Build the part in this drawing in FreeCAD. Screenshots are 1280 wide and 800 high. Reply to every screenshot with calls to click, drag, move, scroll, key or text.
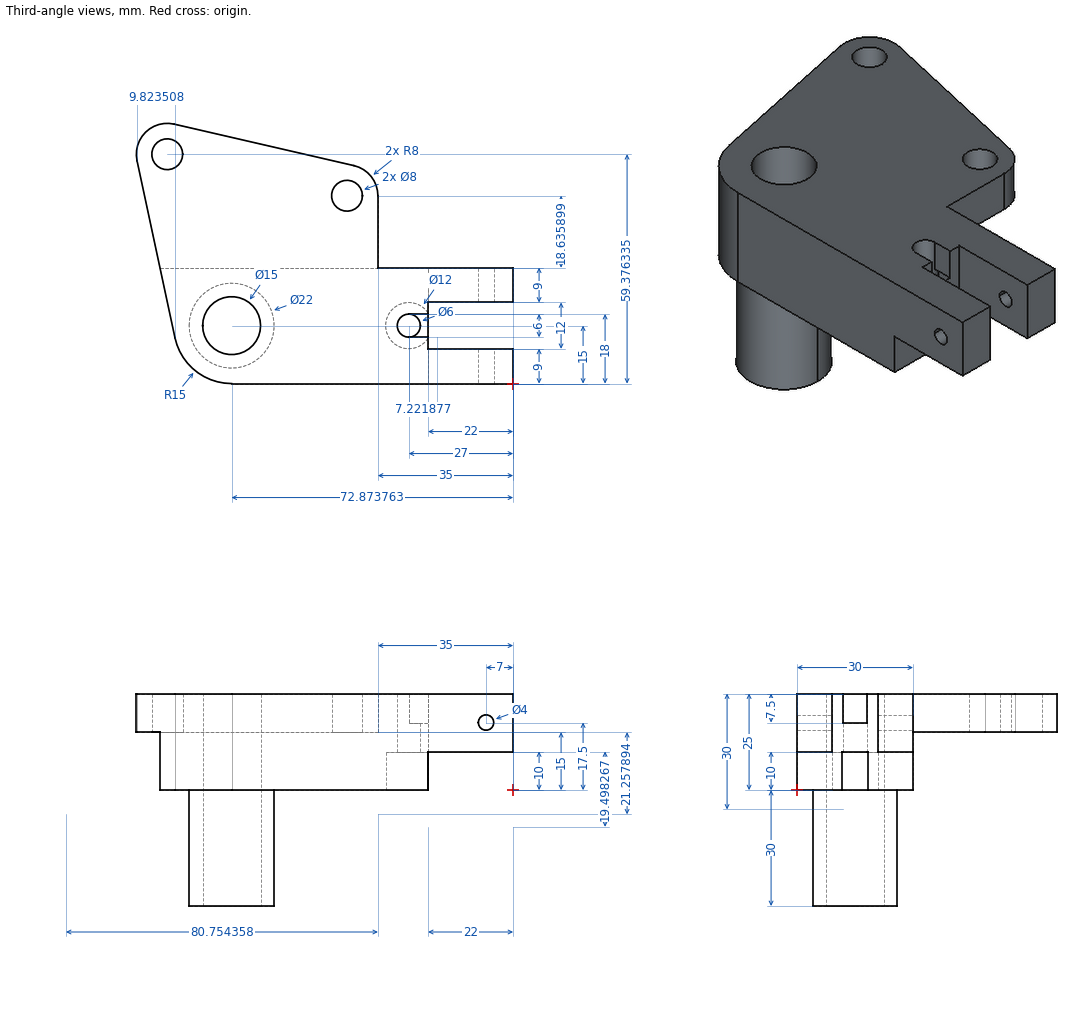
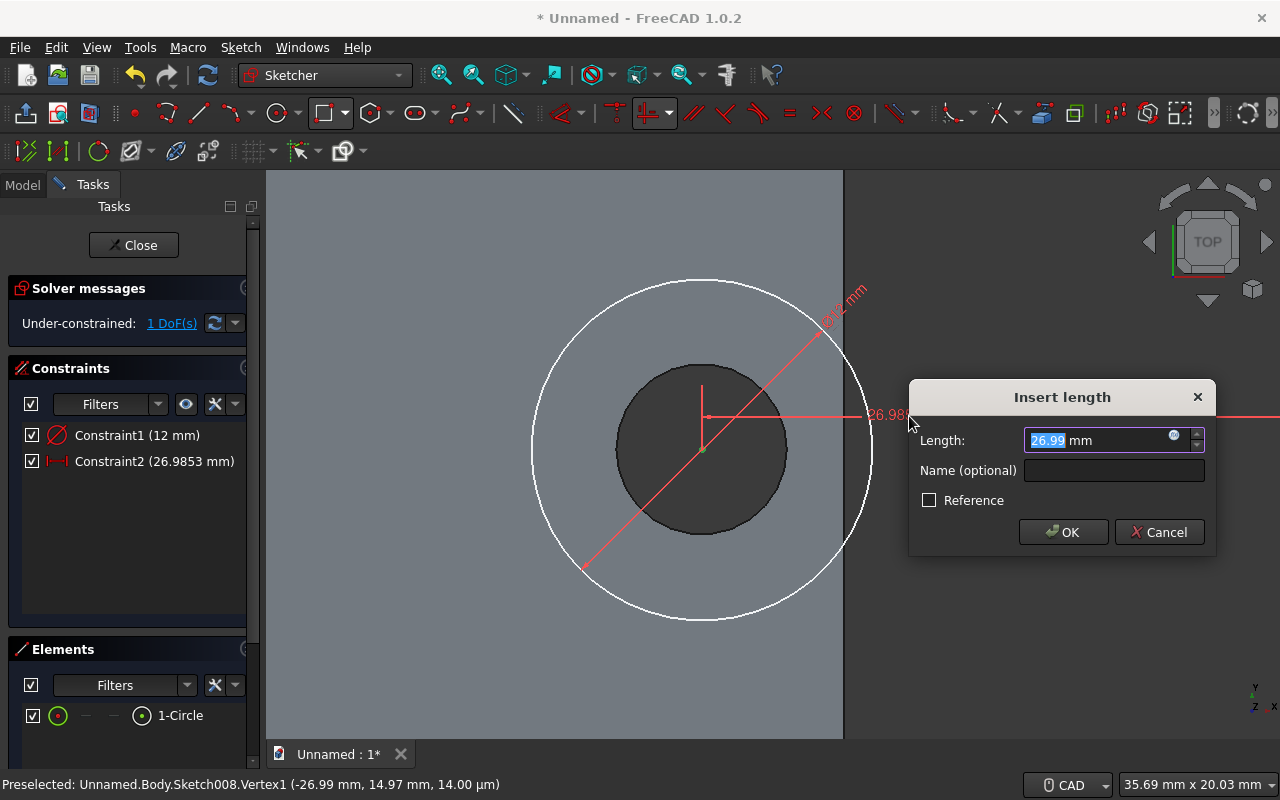
text(27)
key(Return)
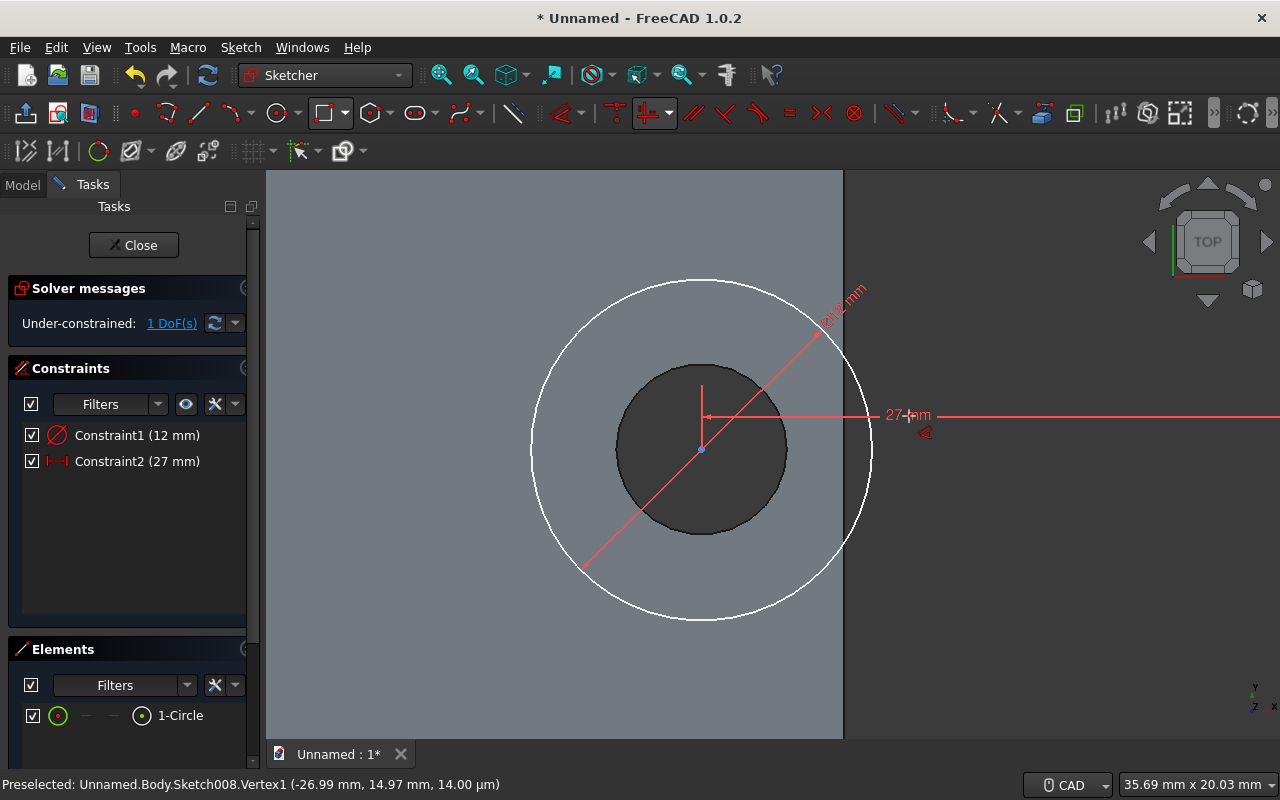
click(702, 450)
click(668, 581)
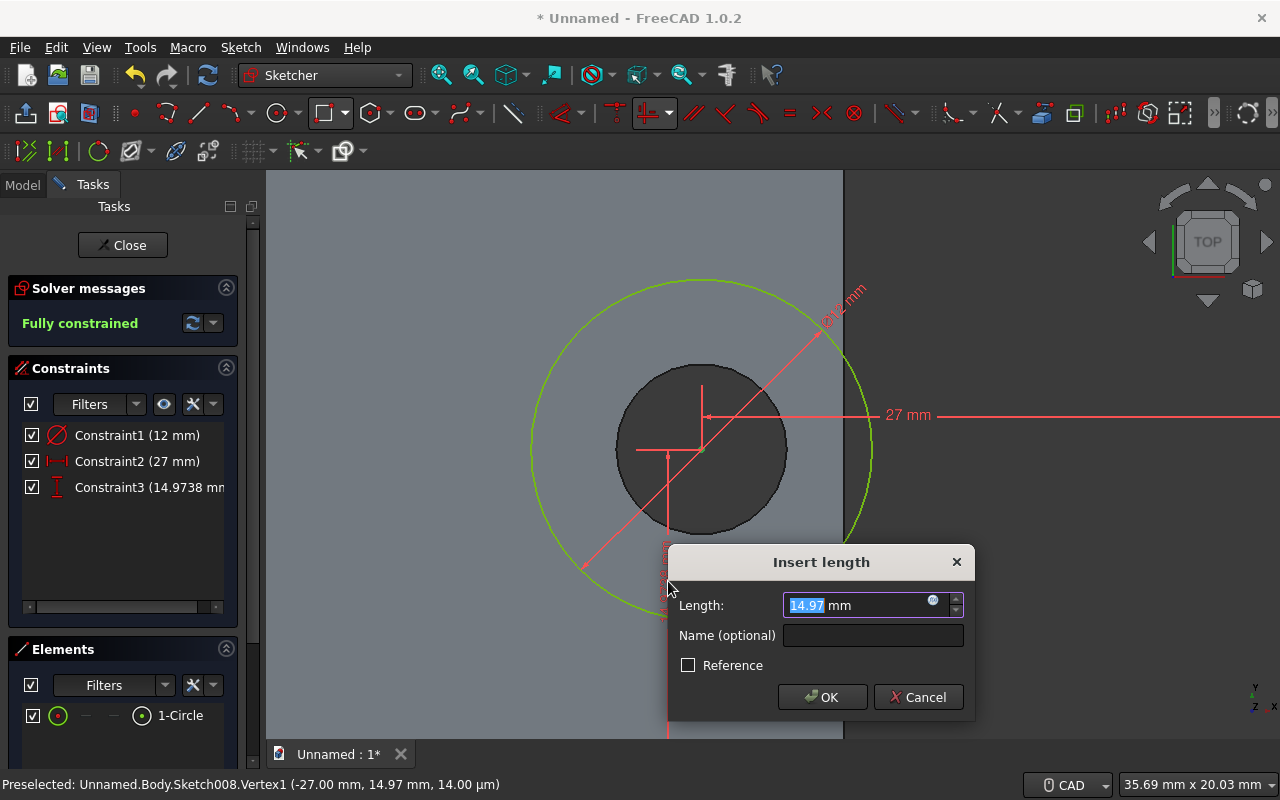
text(15)
key(Return)
key(Escape)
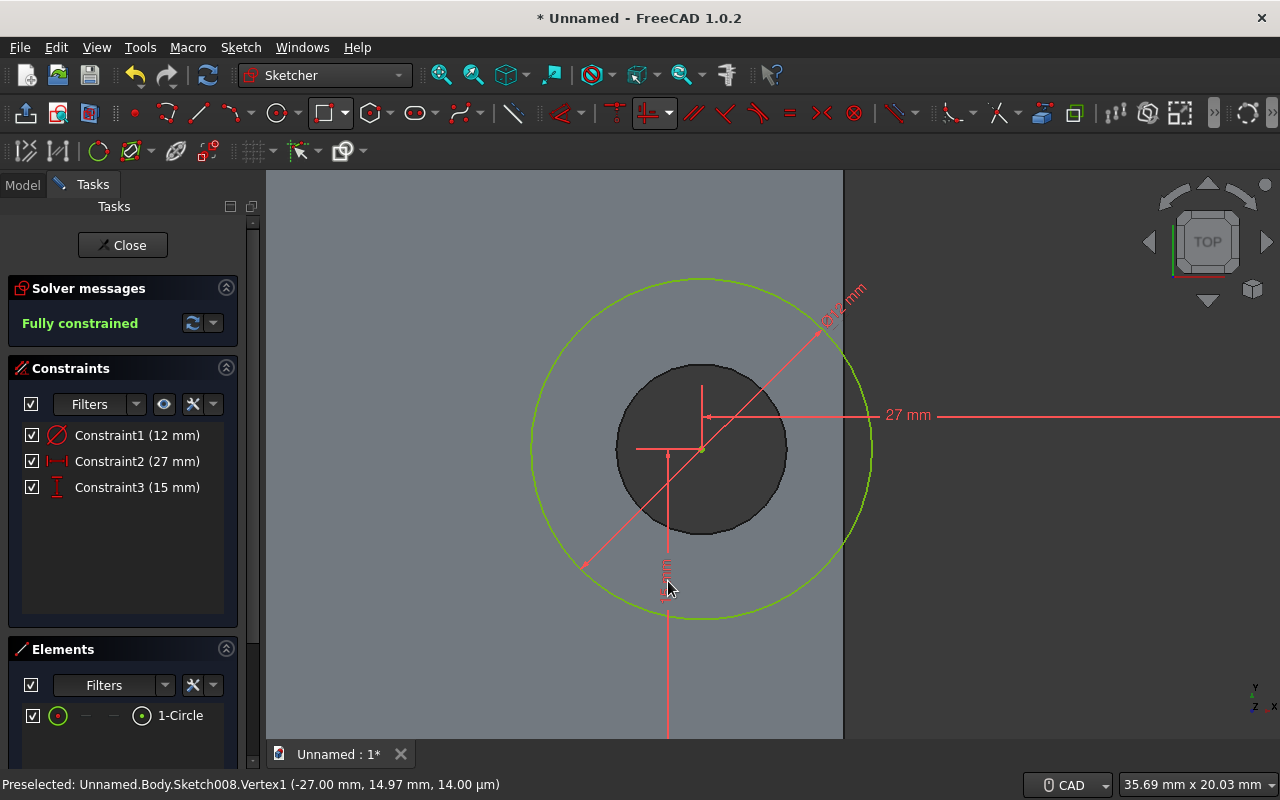
click(123, 245)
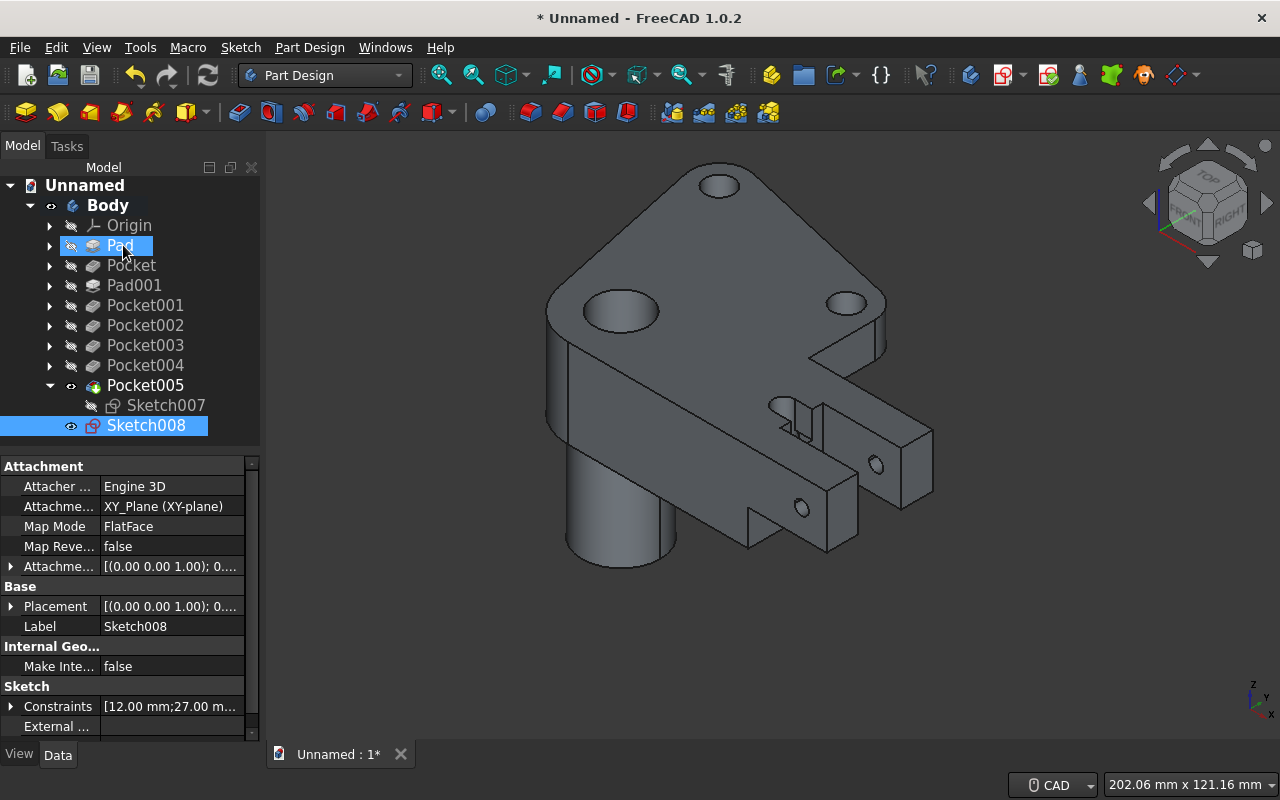
click(240, 112)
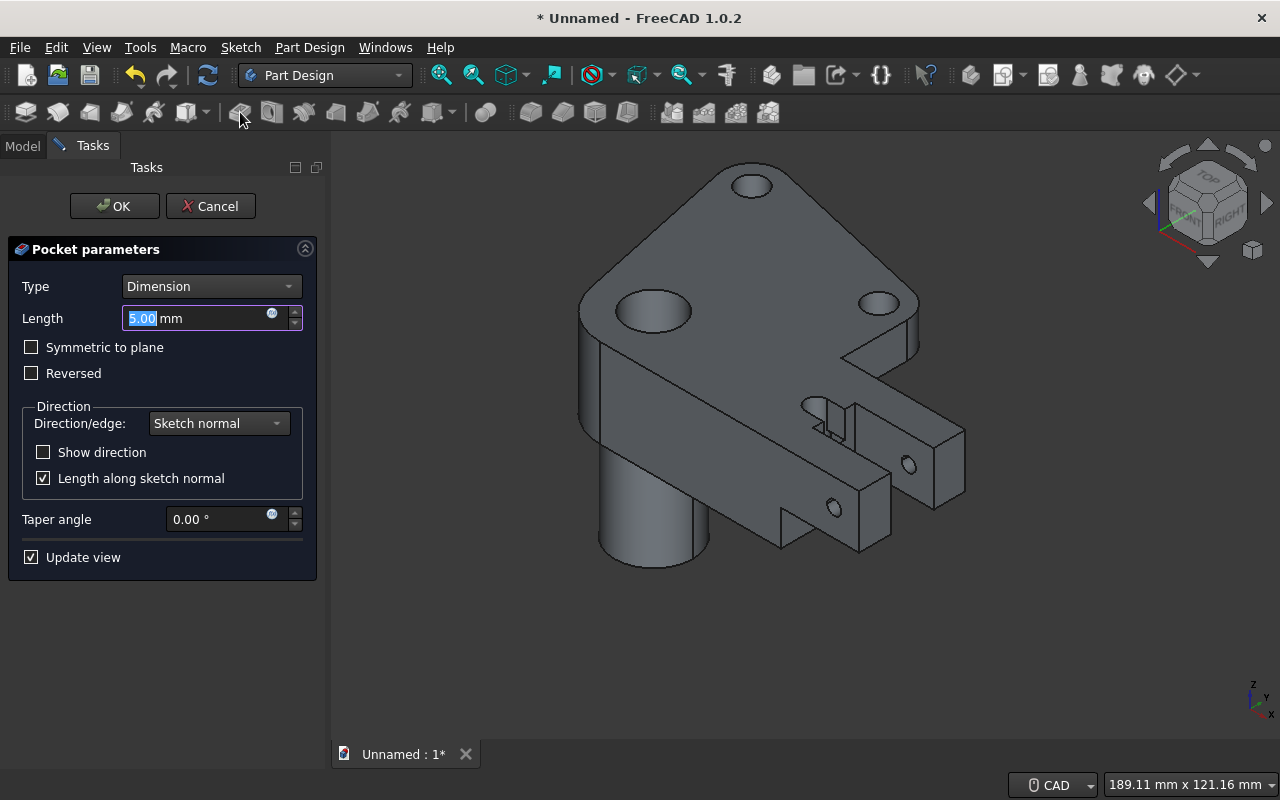
text(10)
key(Tab)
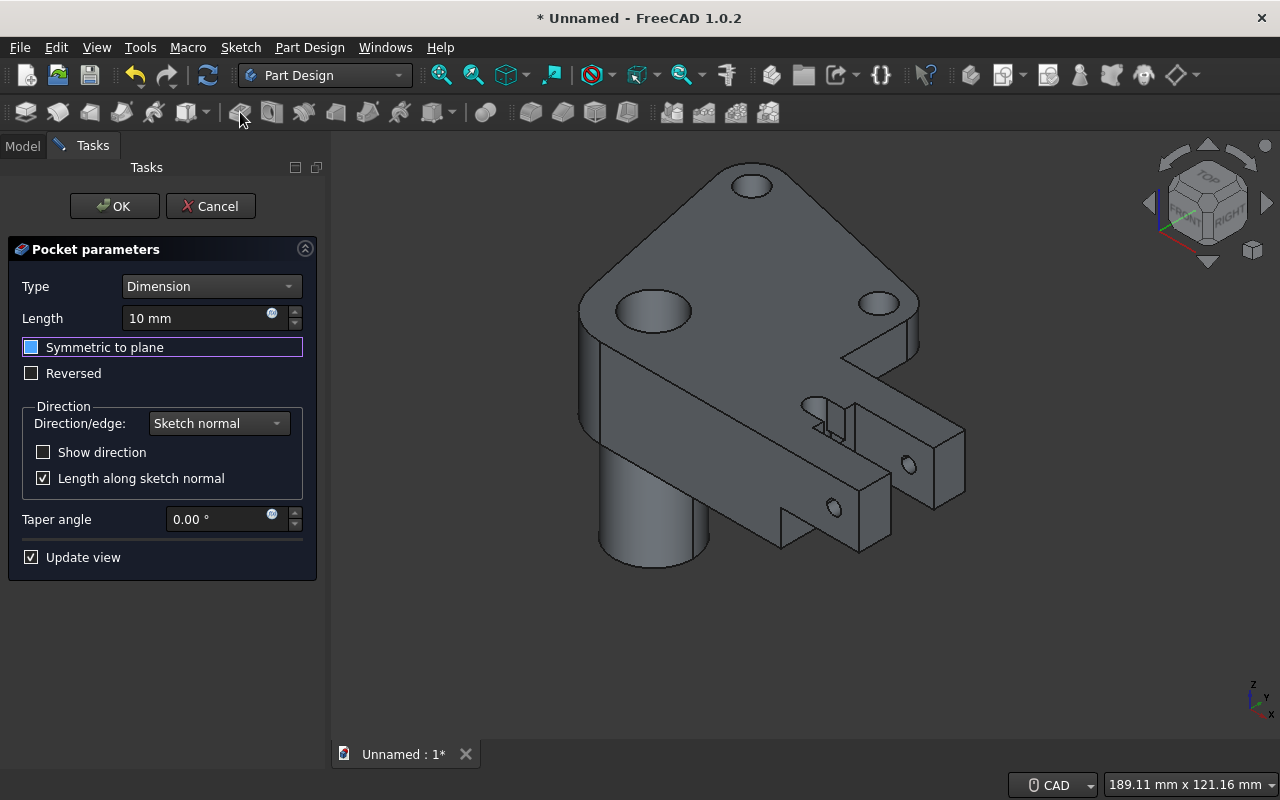
click(30, 373)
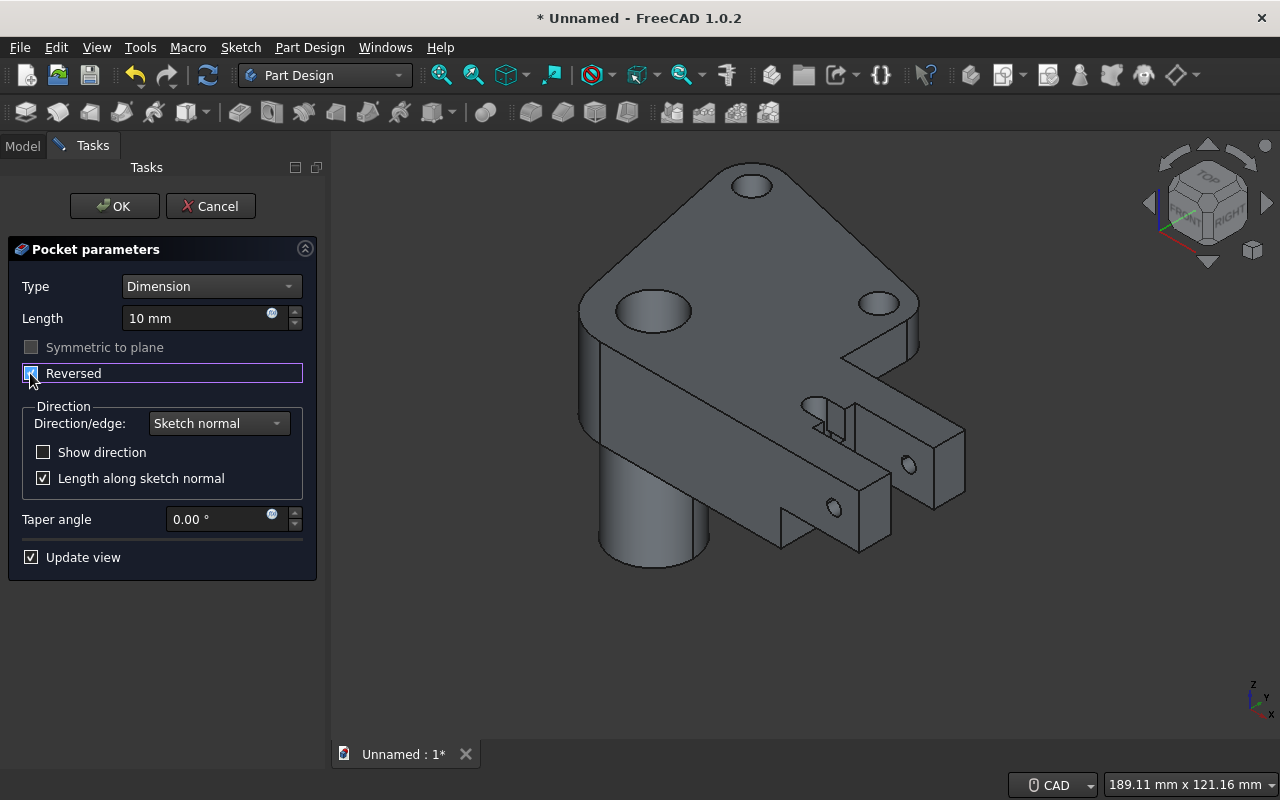
click(115, 206)